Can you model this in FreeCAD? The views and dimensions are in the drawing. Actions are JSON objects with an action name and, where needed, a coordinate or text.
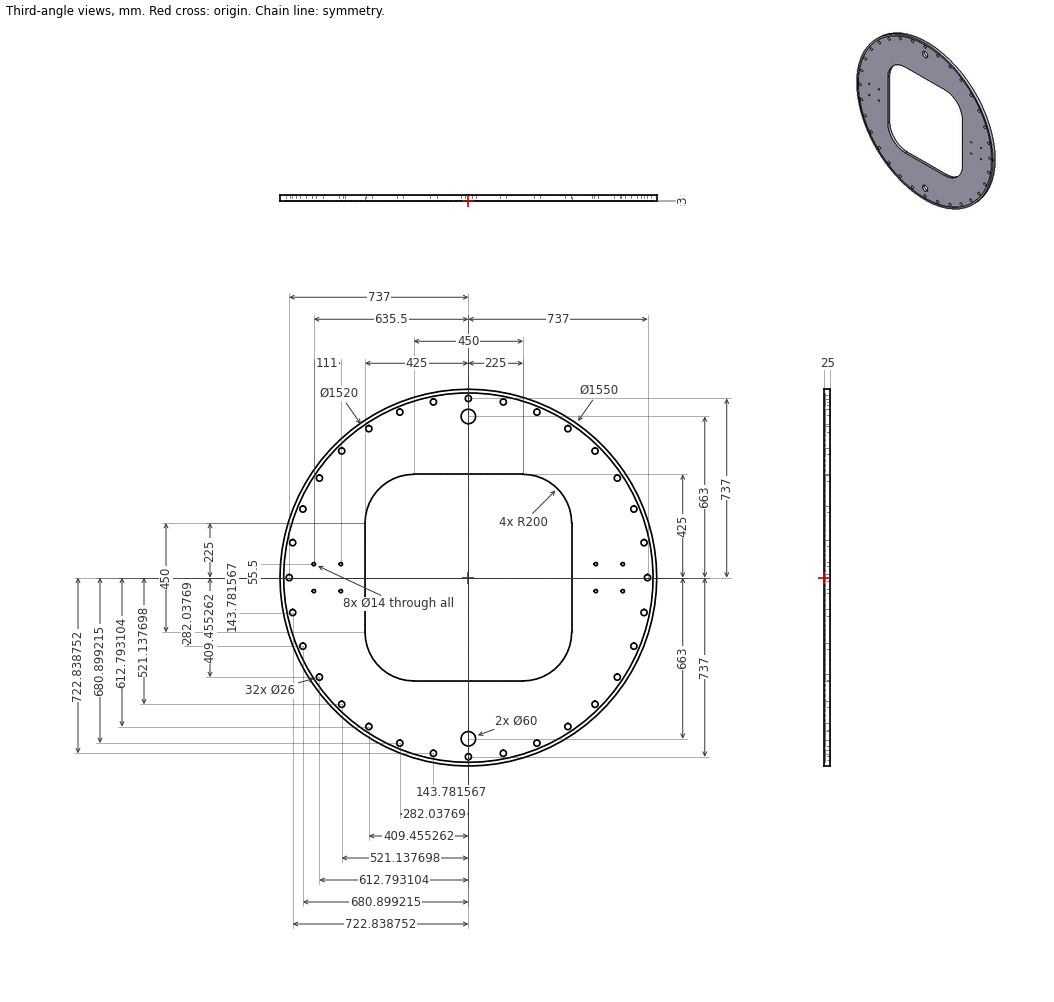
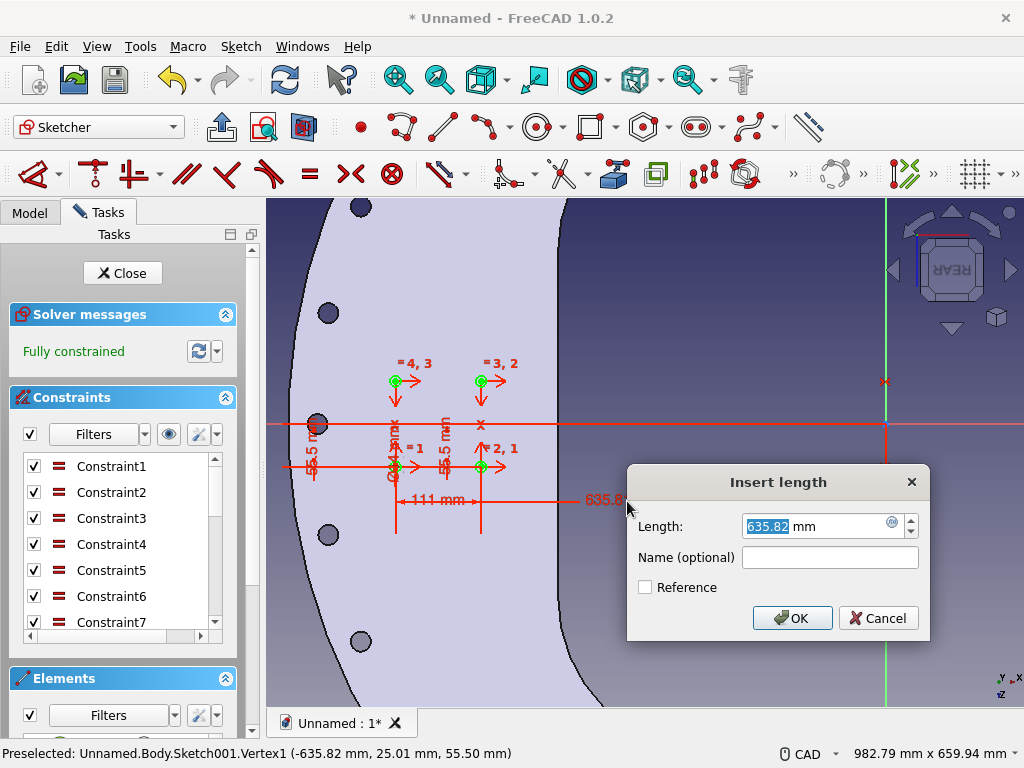
{"action": "type", "text": "635.5"}
{"action": "key", "text": "Return"}
{"action": "key", "text": "Escape"}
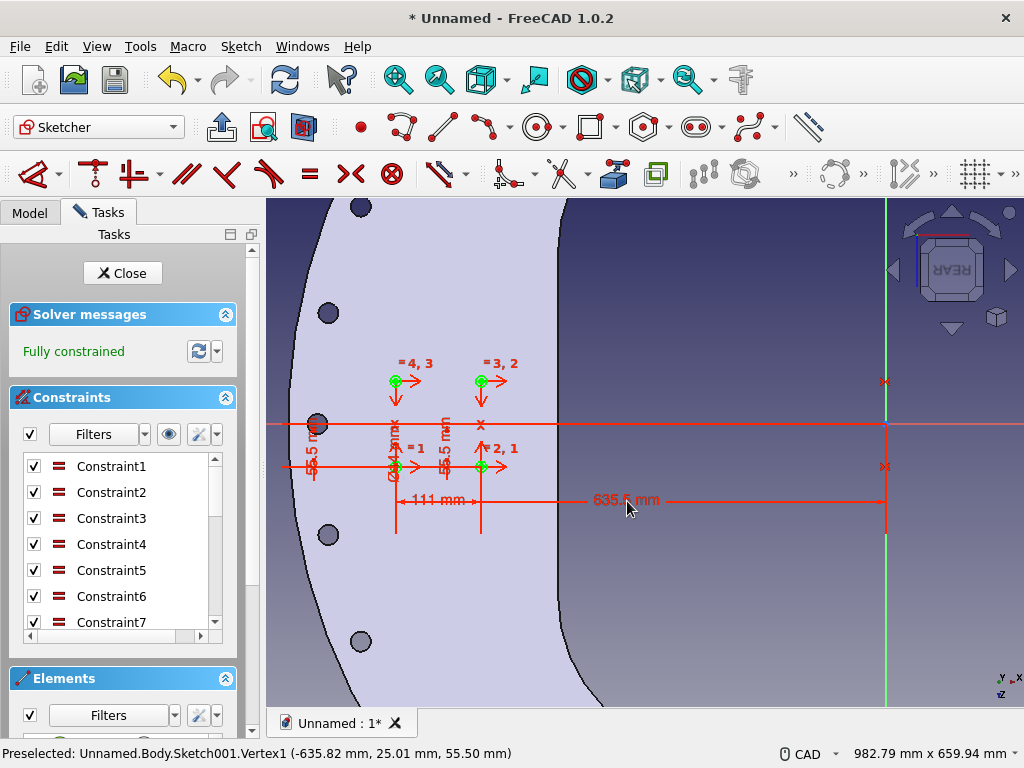
{"action": "left_click", "coordinate": [123, 273]}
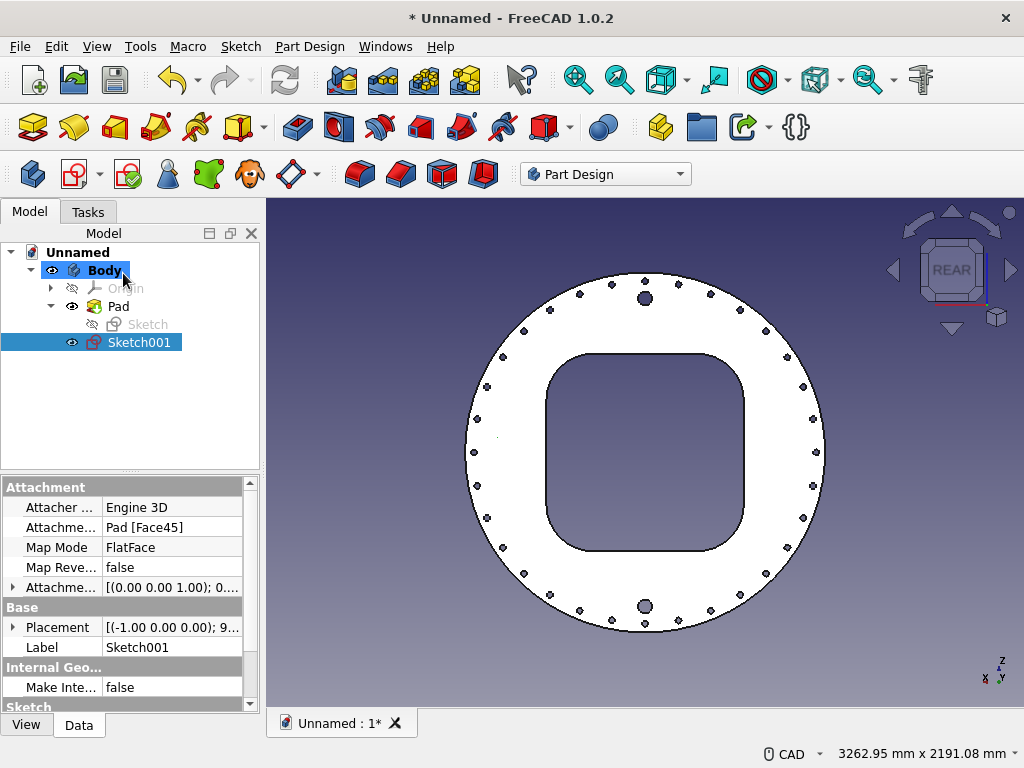
{"action": "left_click", "coordinate": [339, 128]}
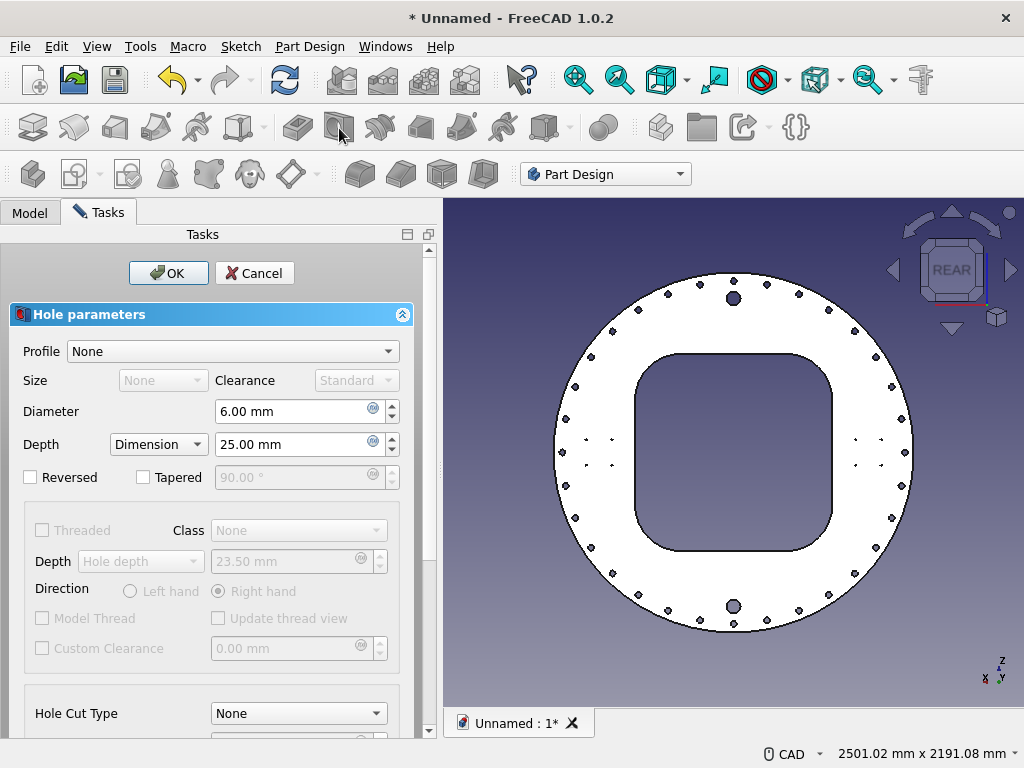
{"action": "triple_click", "coordinate": [300, 412]}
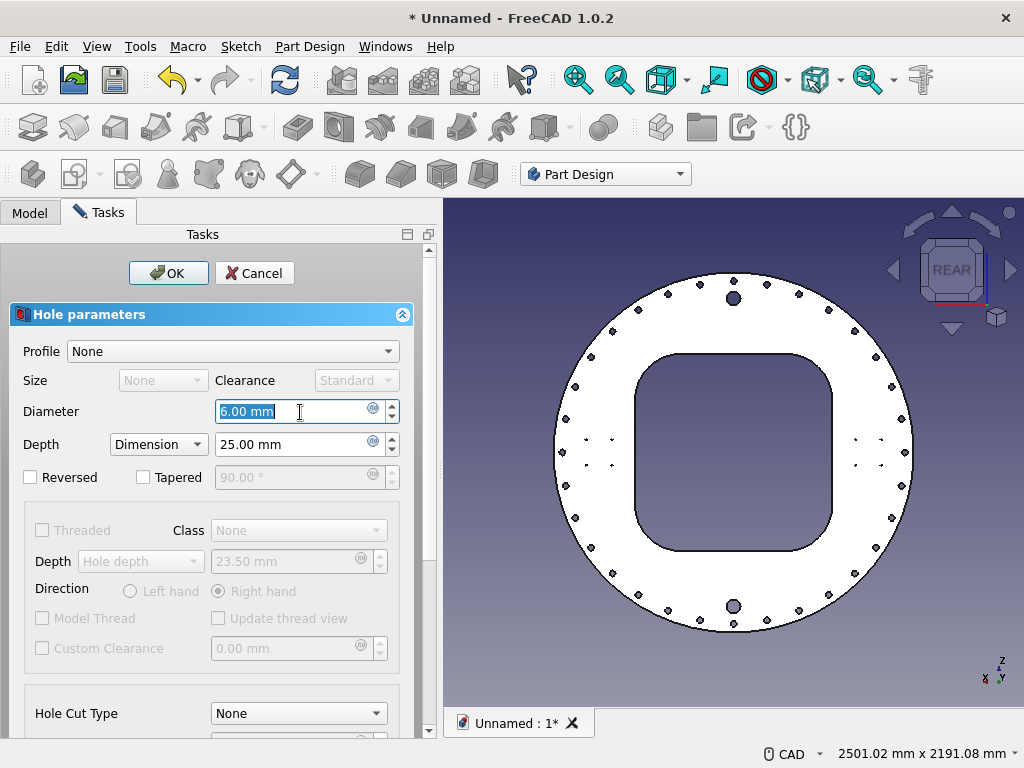
{"action": "type", "text": "14"}
{"action": "key", "text": "Tab"}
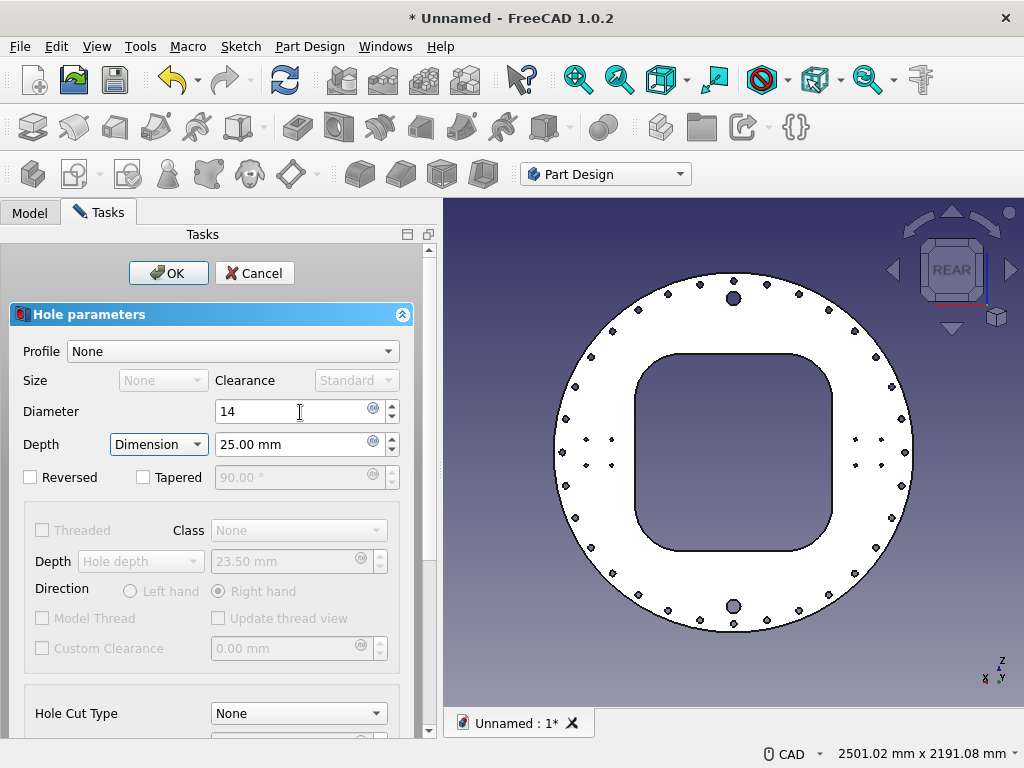
{"action": "left_click", "coordinate": [160, 444]}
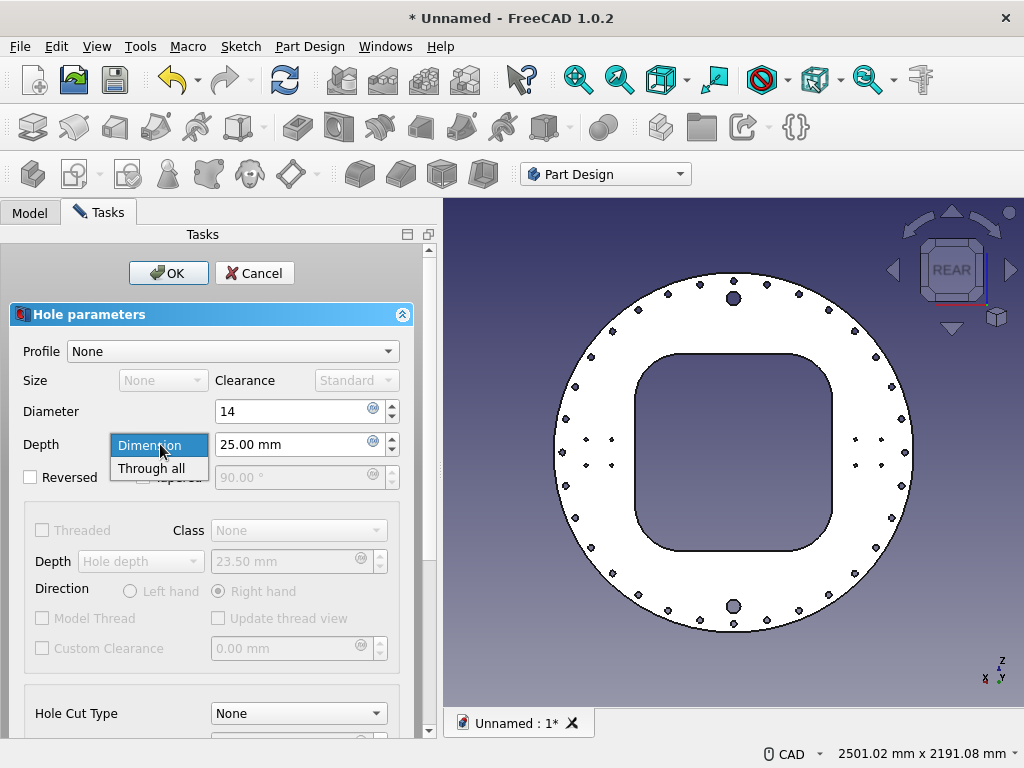
{"action": "left_click", "coordinate": [158, 468]}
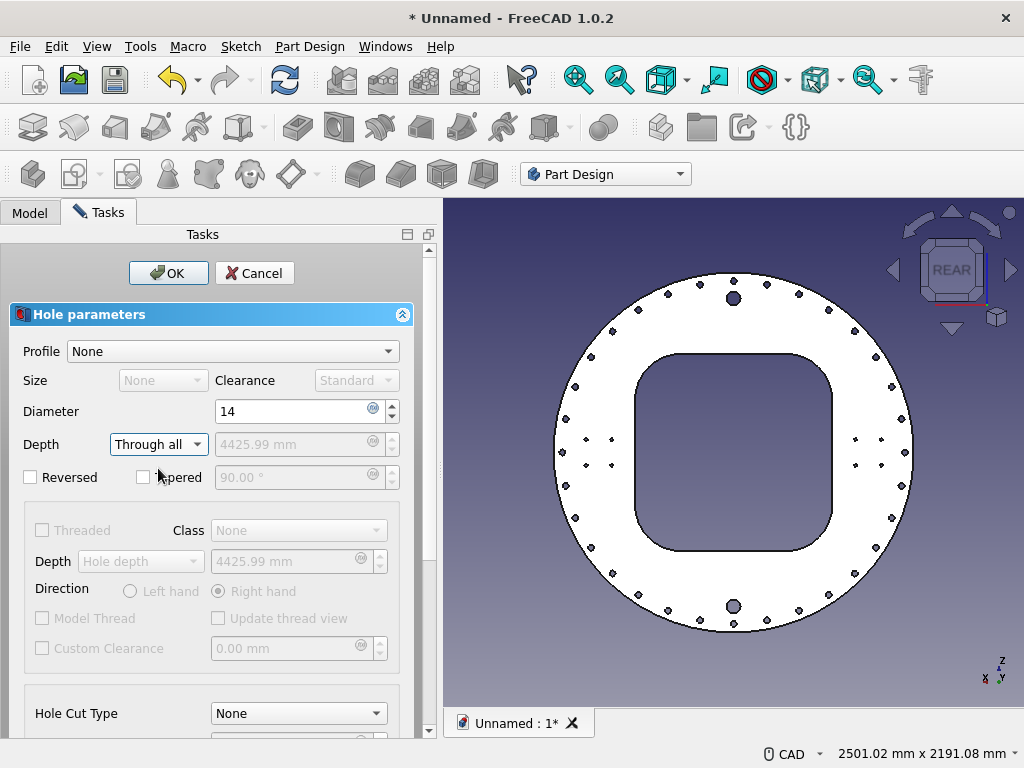
{"action": "left_click", "coordinate": [169, 273]}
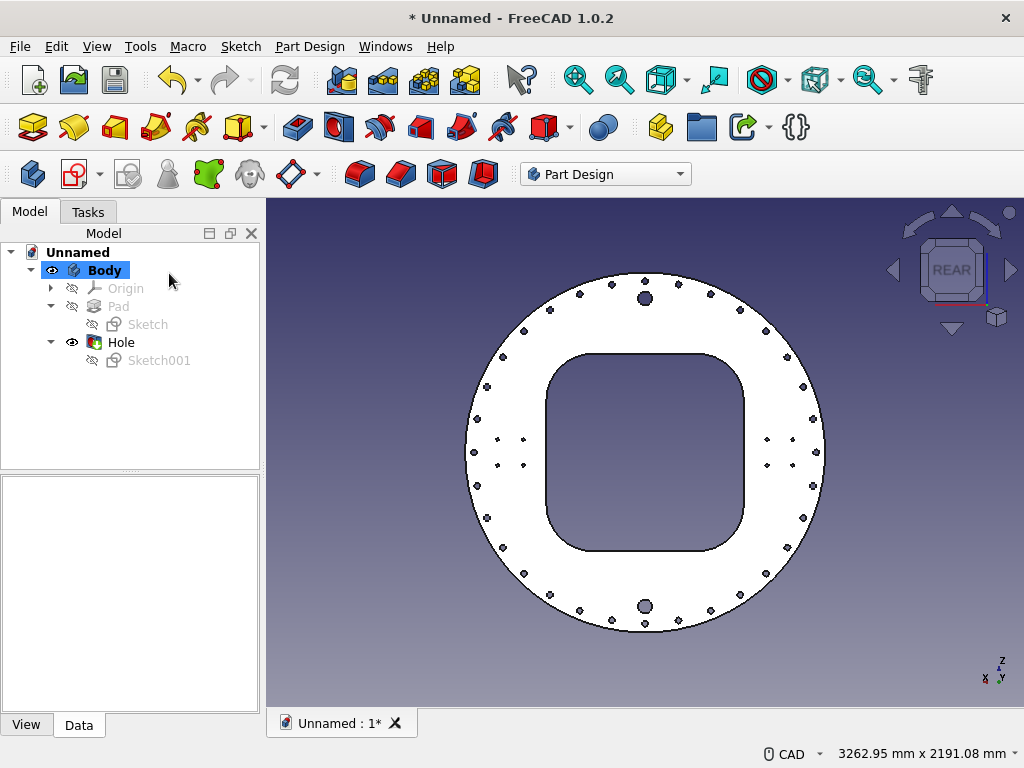
{"action": "left_click", "coordinate": [74, 174]}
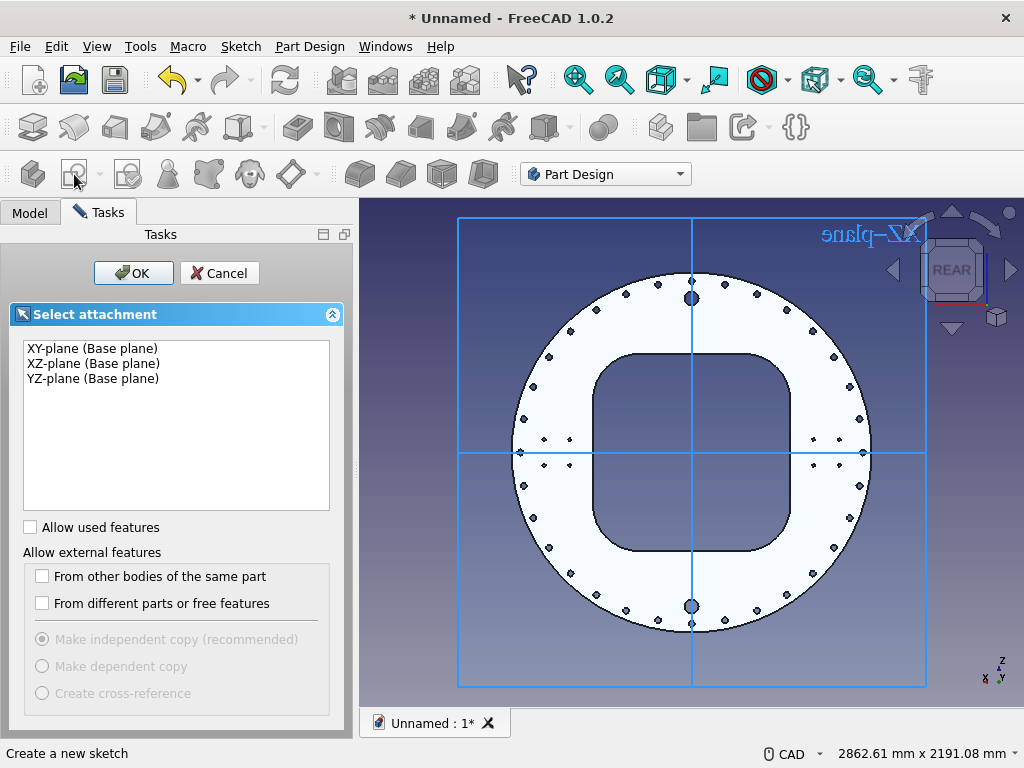
{"action": "left_click", "coordinate": [84, 364]}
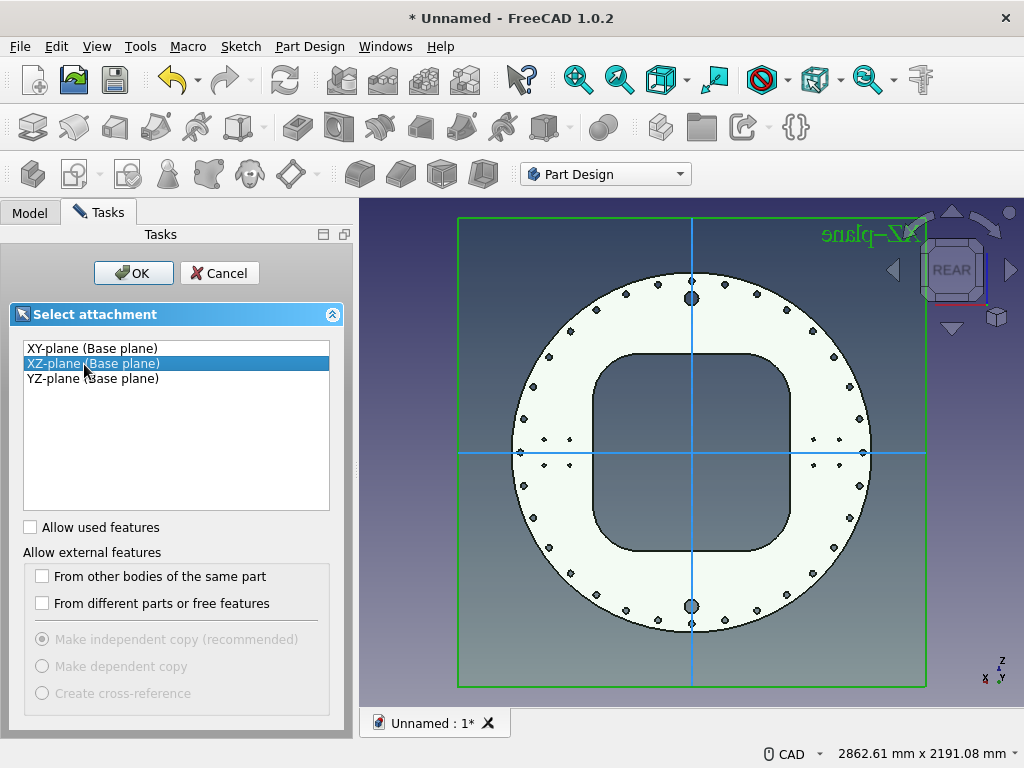
{"action": "left_click", "coordinate": [134, 273]}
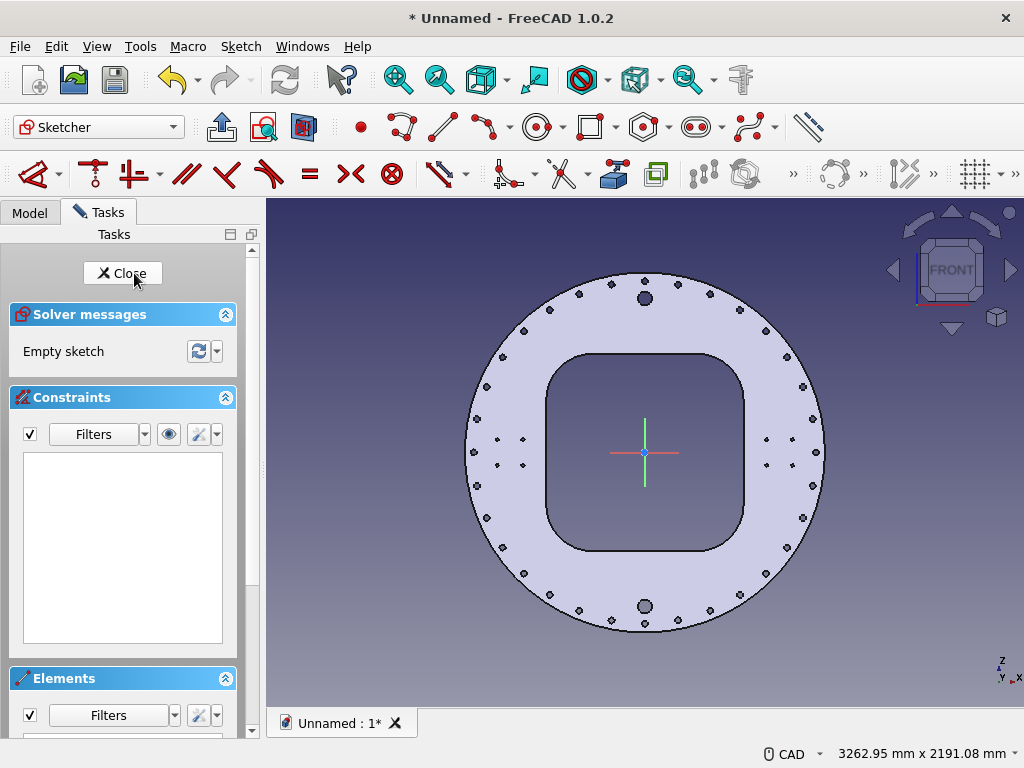
{"action": "left_click", "coordinate": [536, 128]}